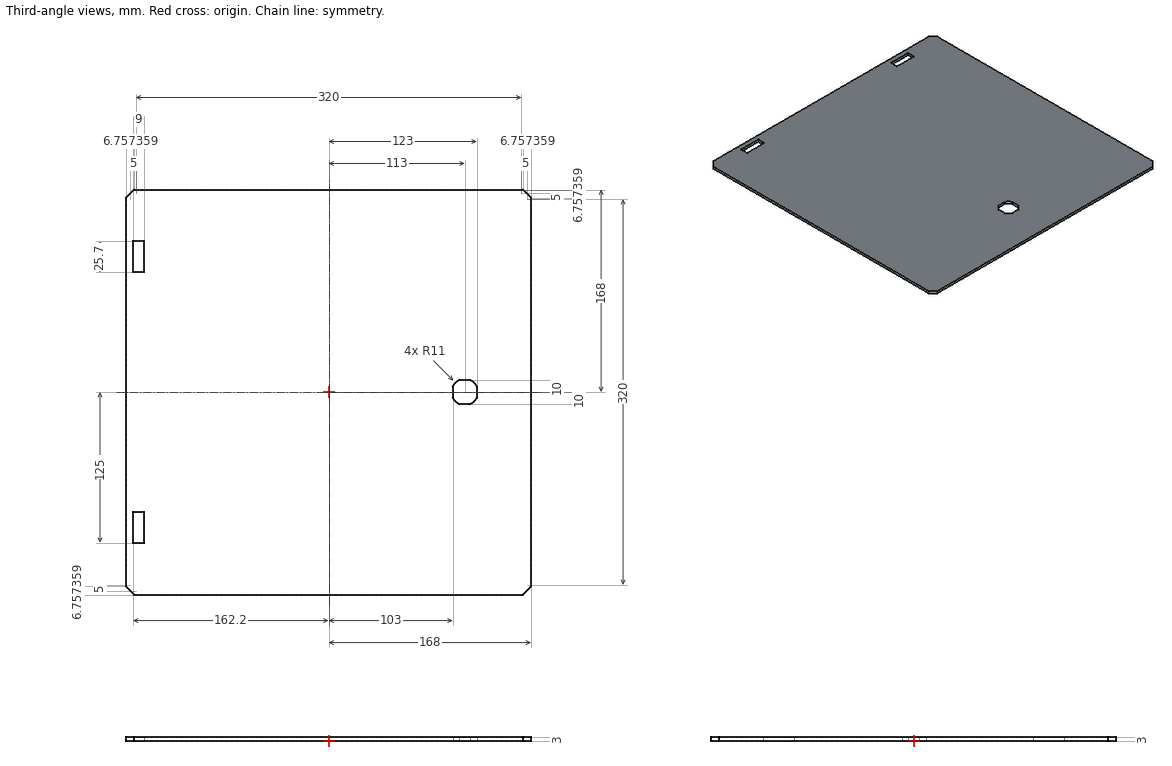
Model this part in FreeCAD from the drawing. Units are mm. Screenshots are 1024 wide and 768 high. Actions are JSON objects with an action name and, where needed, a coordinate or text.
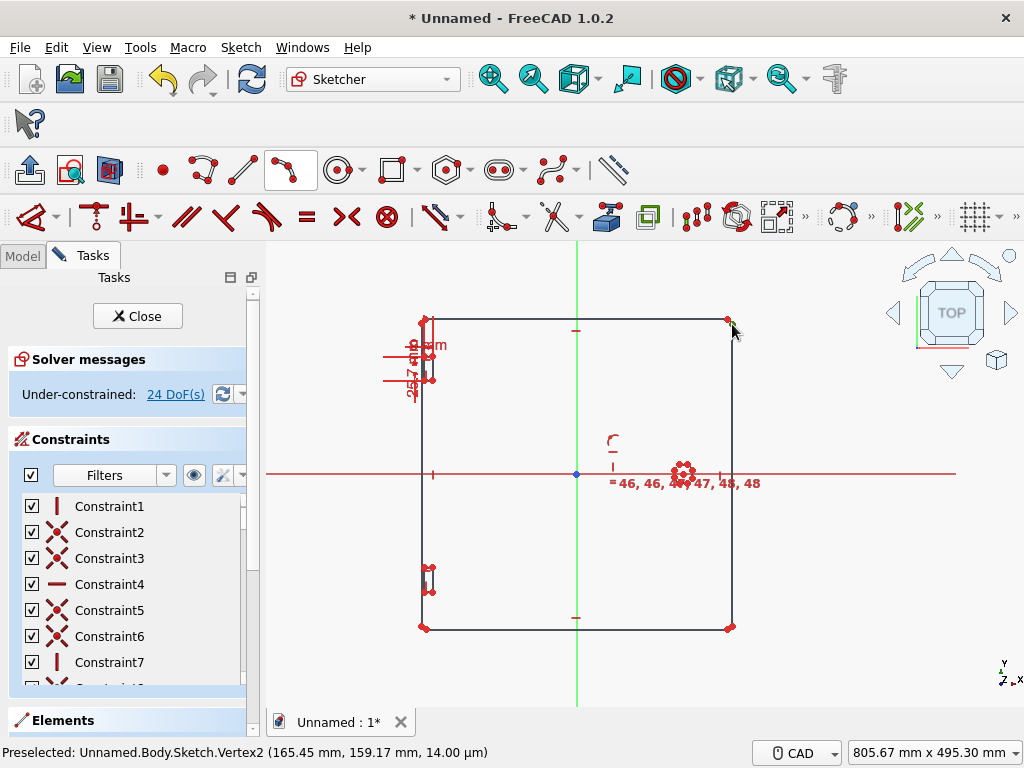
{"action": "scroll", "coordinate": [422, 324], "scroll_direction": "up", "scroll_amount": 4}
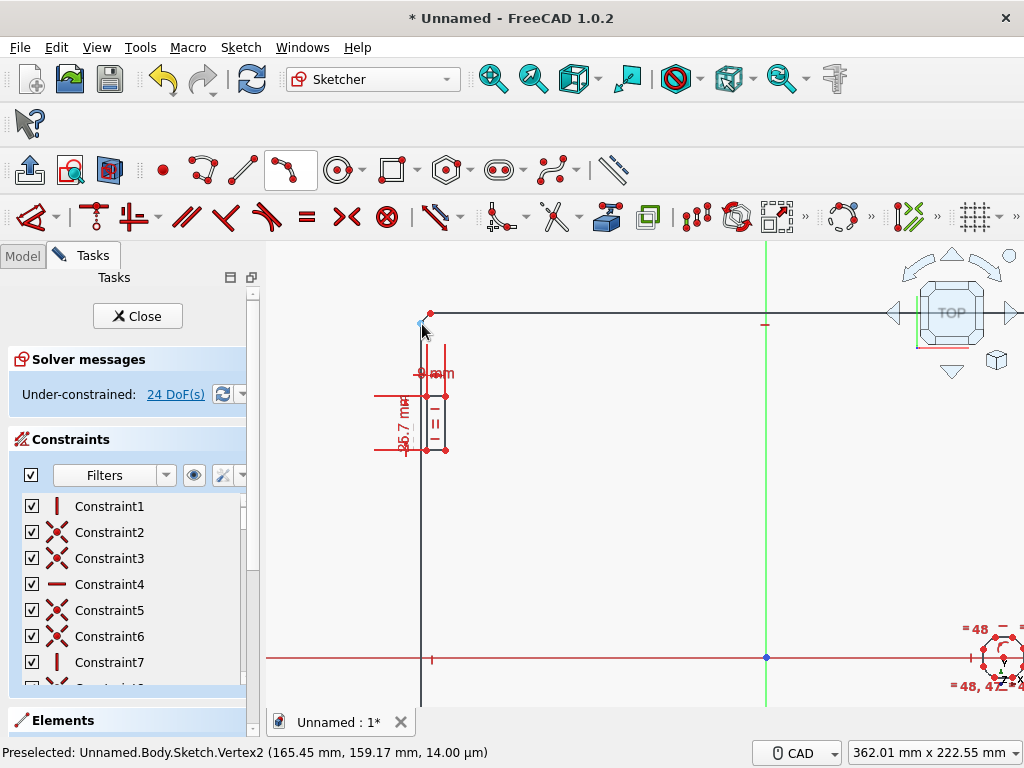
{"action": "left_click", "coordinate": [421, 323]}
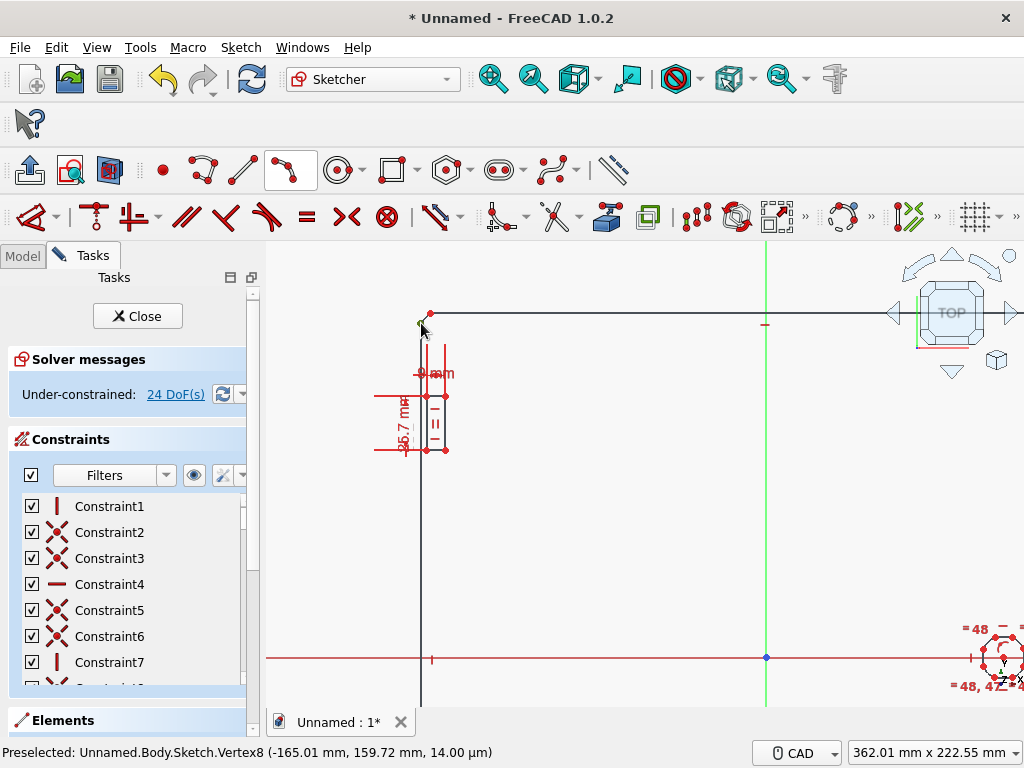
{"action": "left_click", "coordinate": [766, 620]}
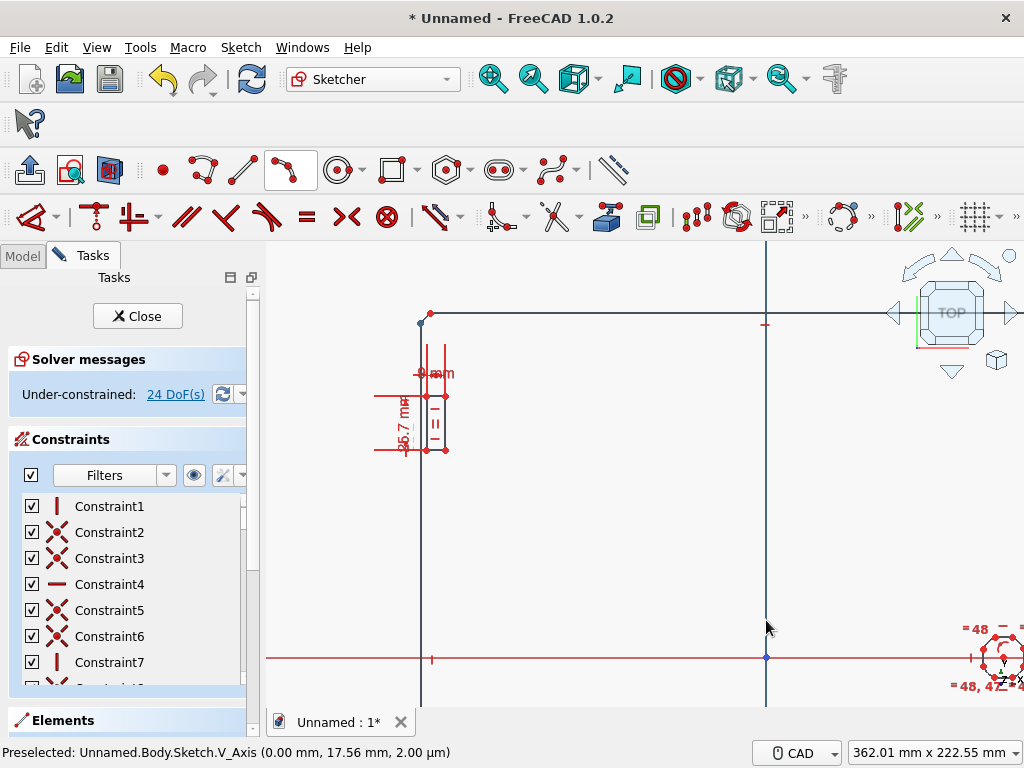
{"action": "left_click", "coordinate": [348, 218]}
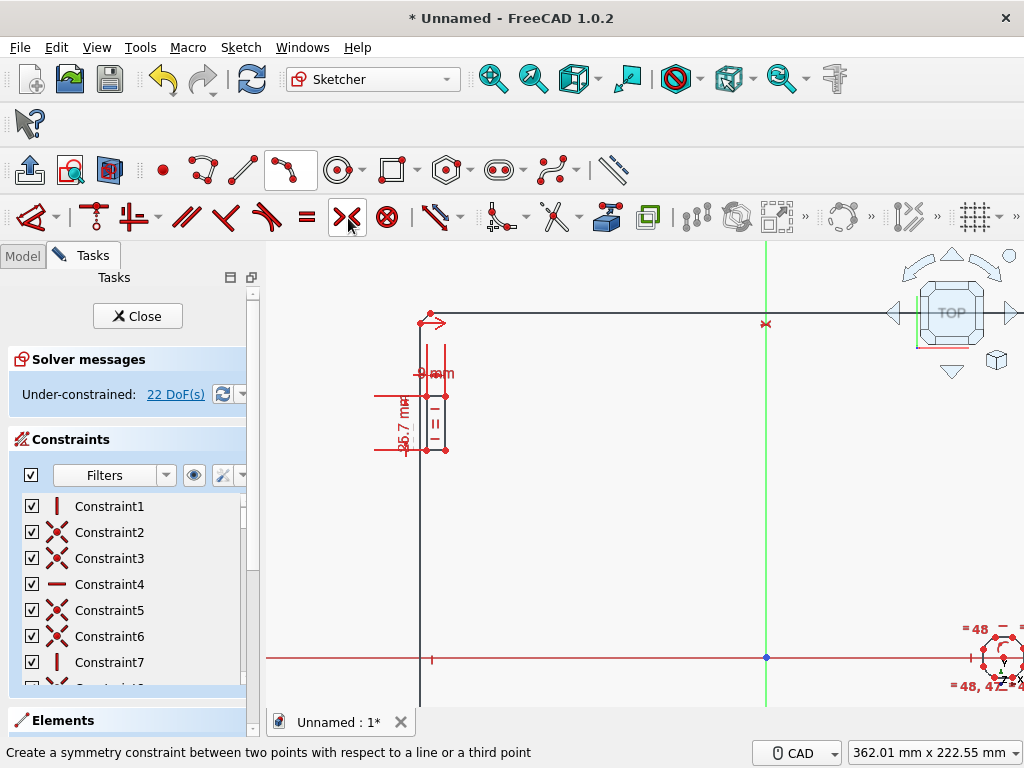
{"action": "left_click", "coordinate": [430, 313]}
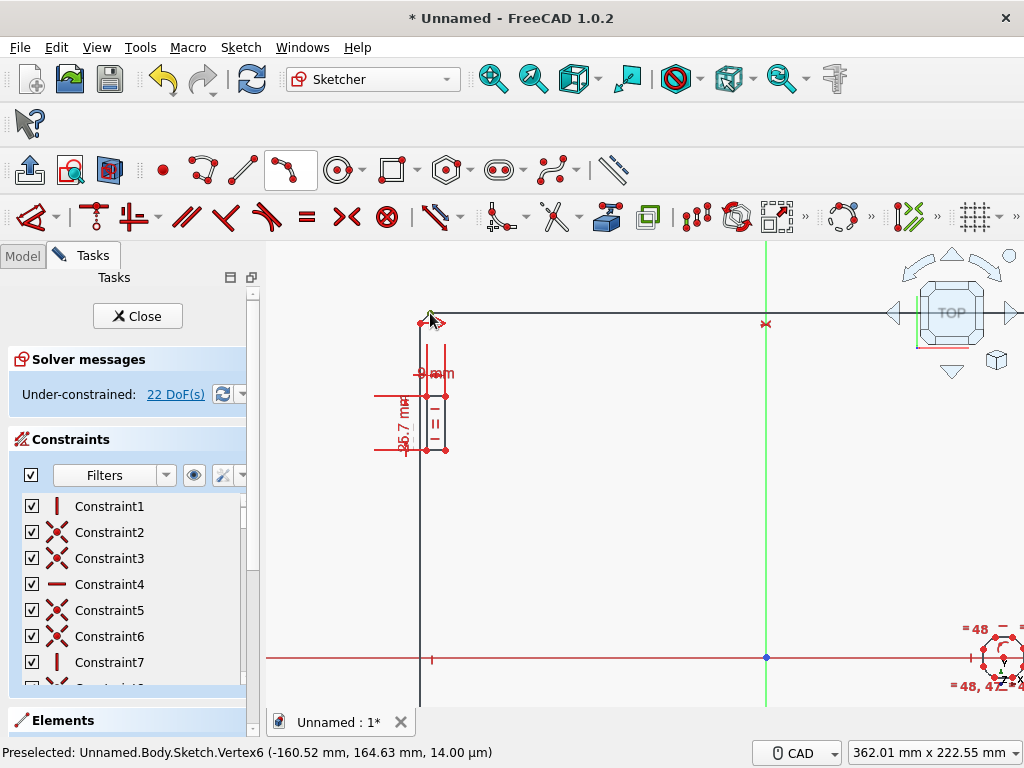
{"action": "scroll", "coordinate": [422, 324], "scroll_direction": "down", "scroll_amount": 4}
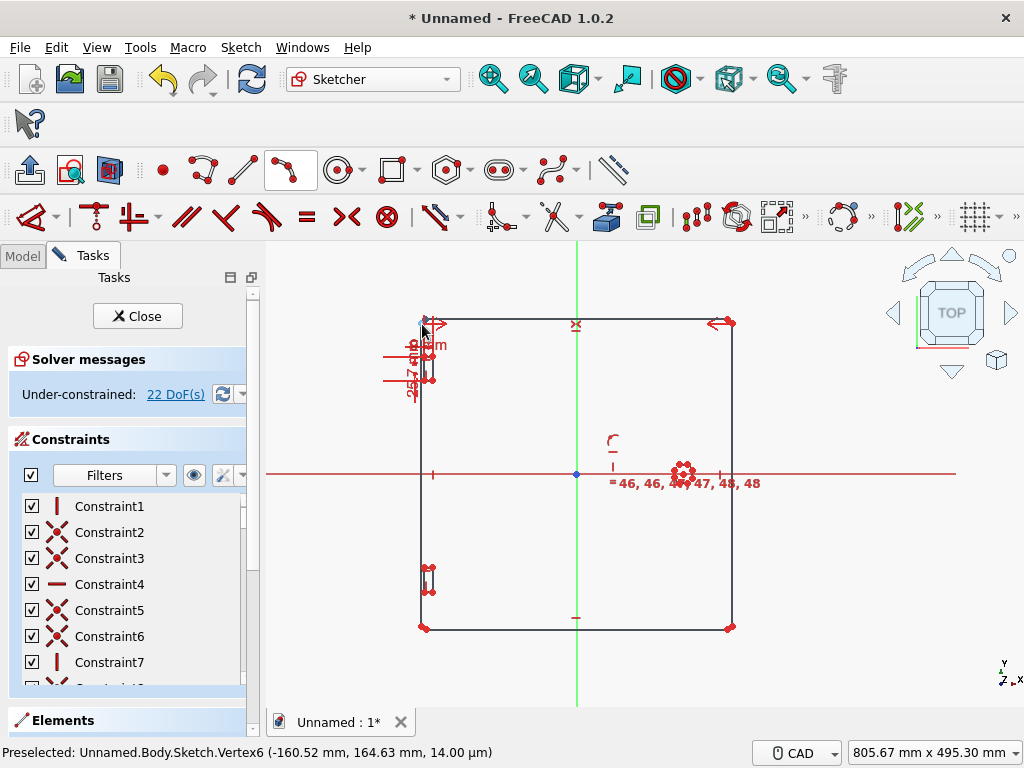
{"action": "scroll", "coordinate": [426, 630], "scroll_direction": "up", "scroll_amount": 4}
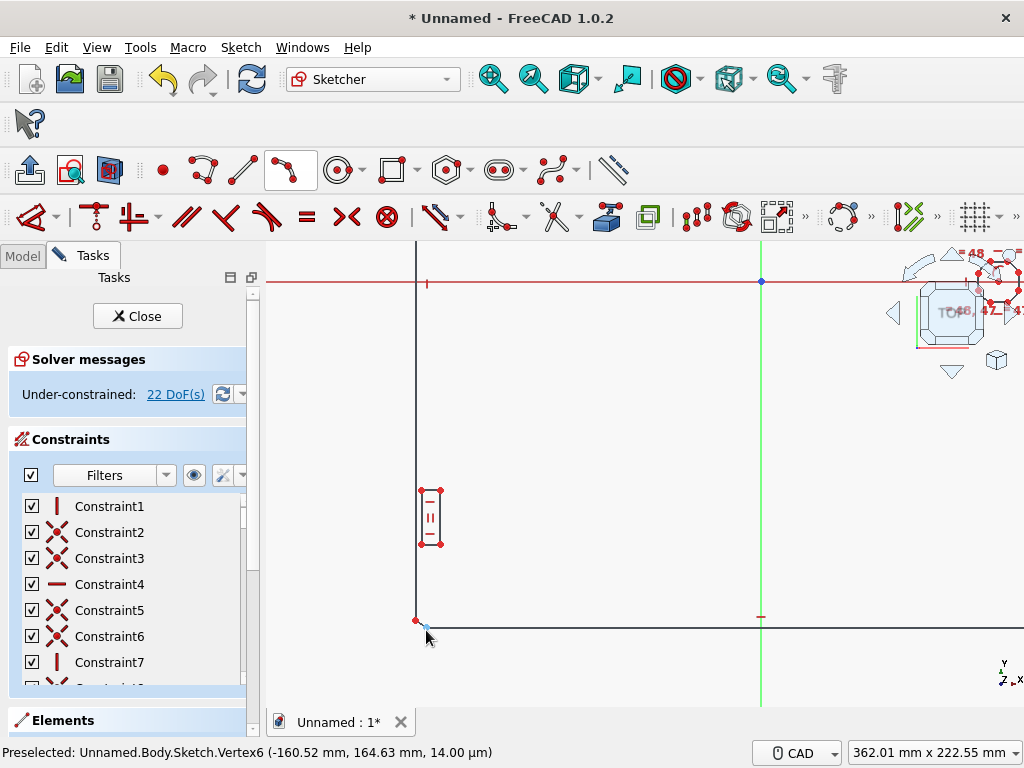
{"action": "left_click", "coordinate": [426, 628]}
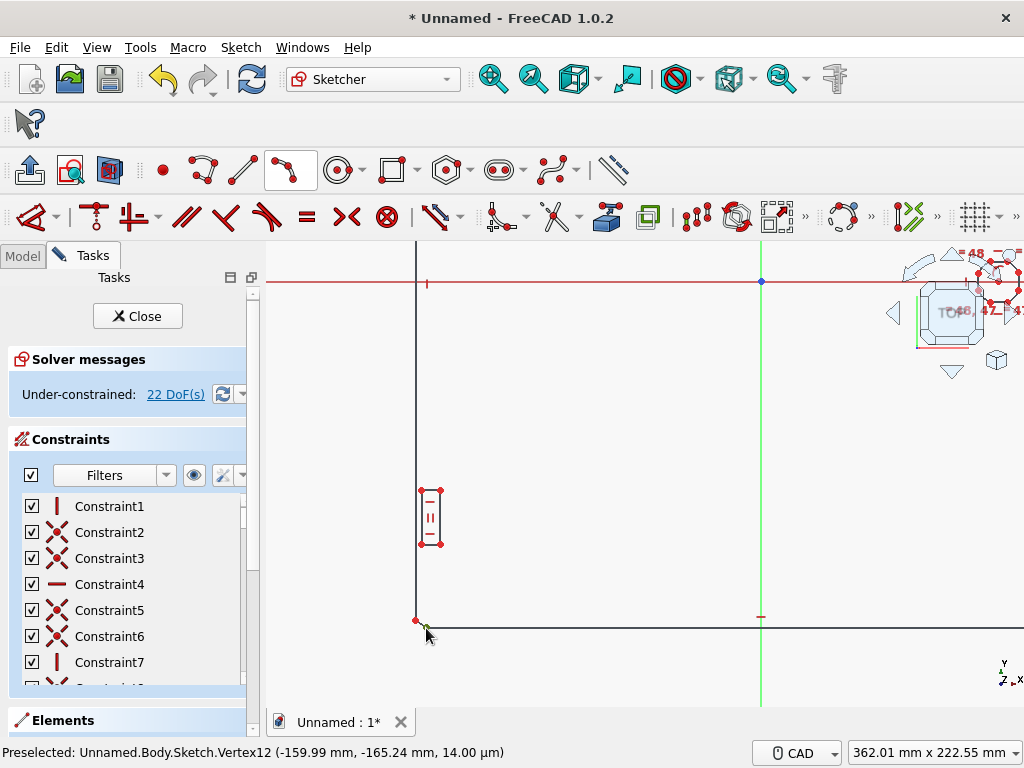
{"action": "left_click", "coordinate": [334, 282]}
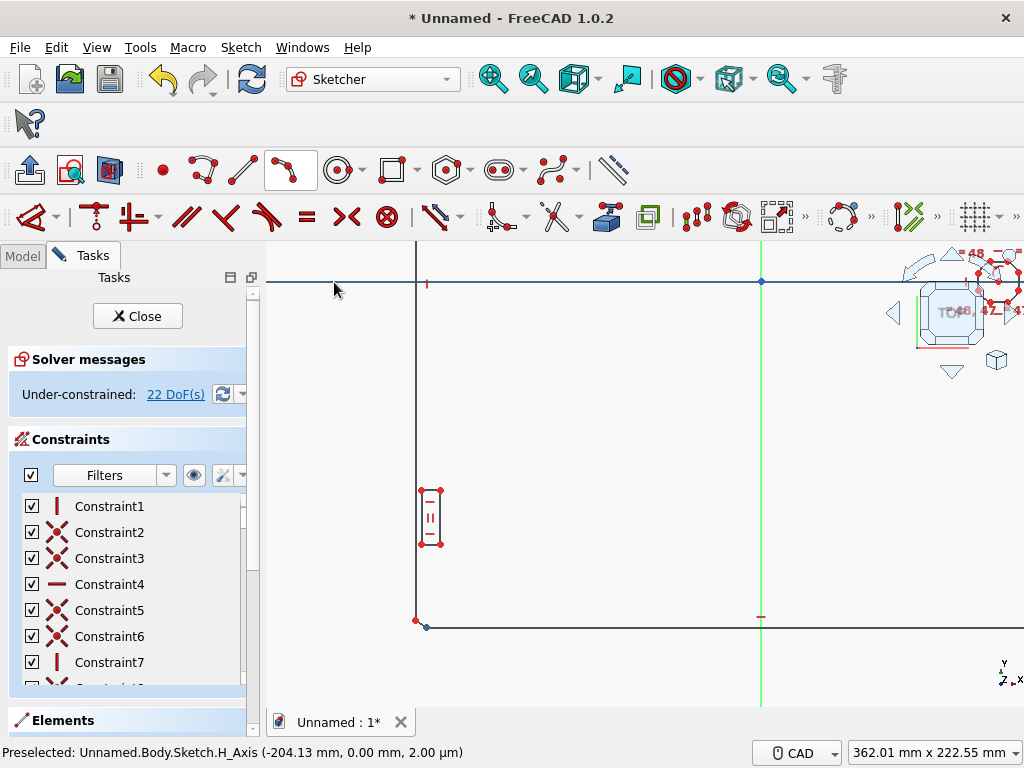
{"action": "left_click", "coordinate": [348, 218]}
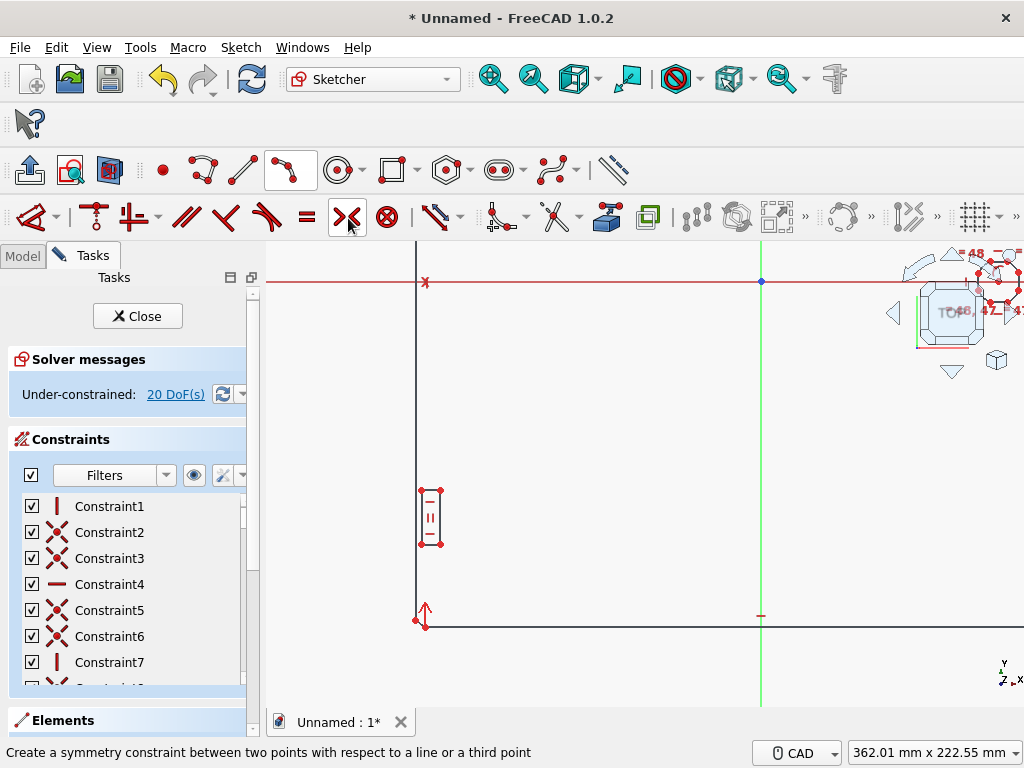
{"action": "left_click", "coordinate": [422, 545]}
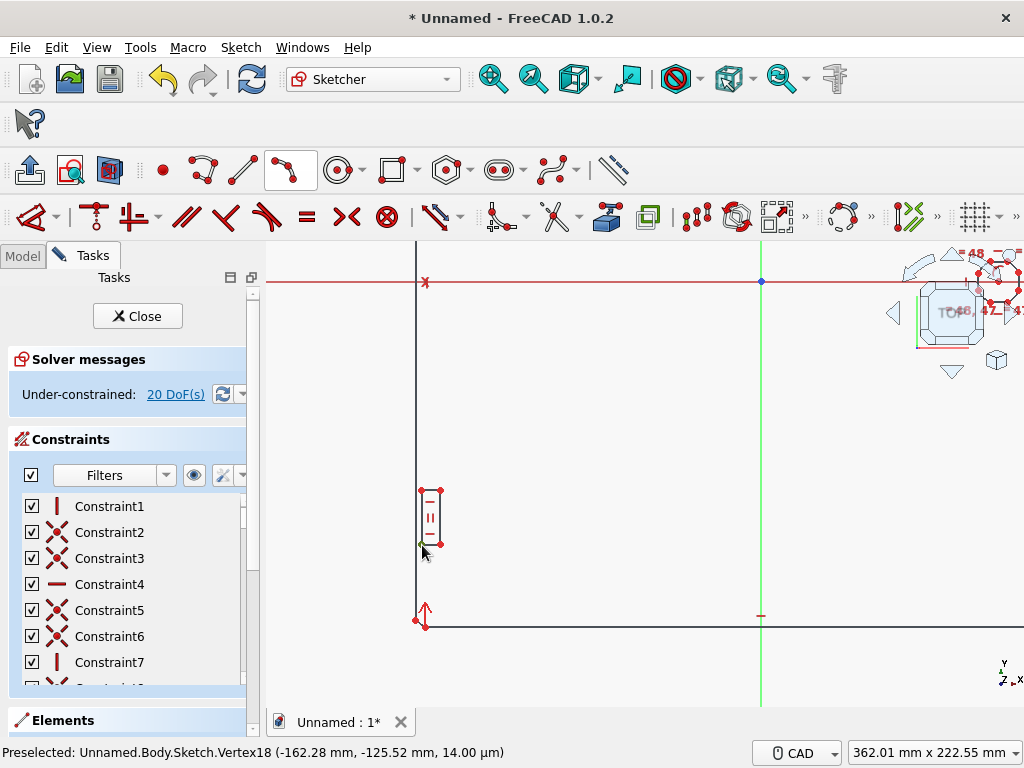
{"action": "scroll", "coordinate": [426, 631], "scroll_direction": "down", "scroll_amount": 4}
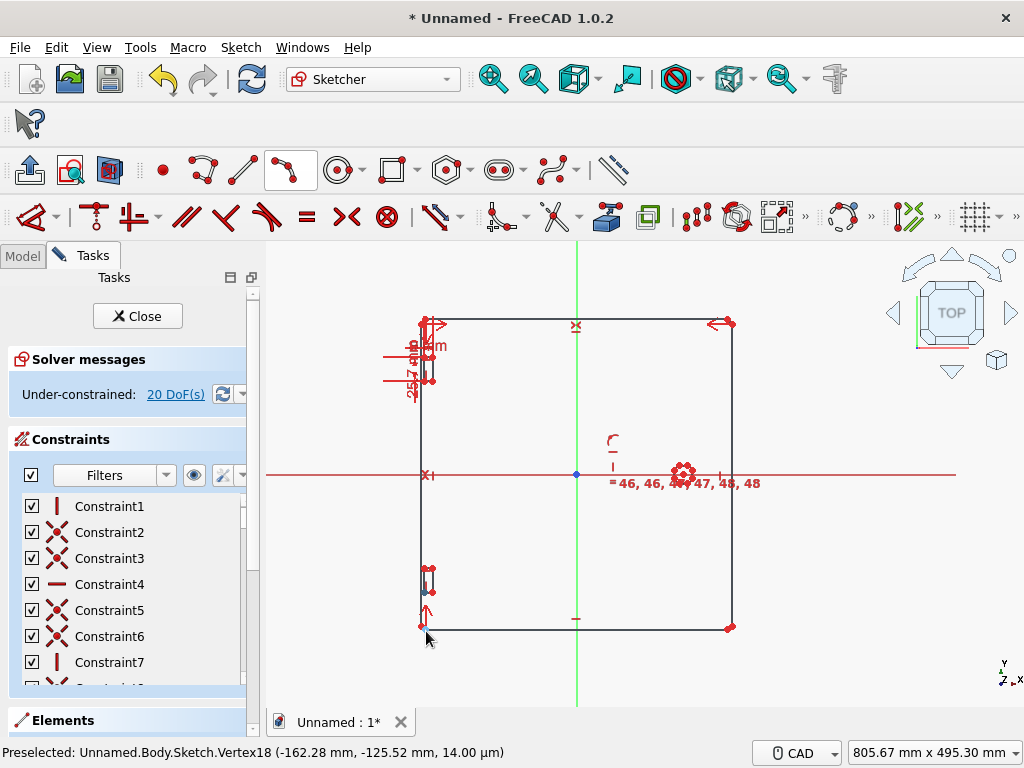
{"action": "scroll", "coordinate": [424, 357], "scroll_direction": "up", "scroll_amount": 2}